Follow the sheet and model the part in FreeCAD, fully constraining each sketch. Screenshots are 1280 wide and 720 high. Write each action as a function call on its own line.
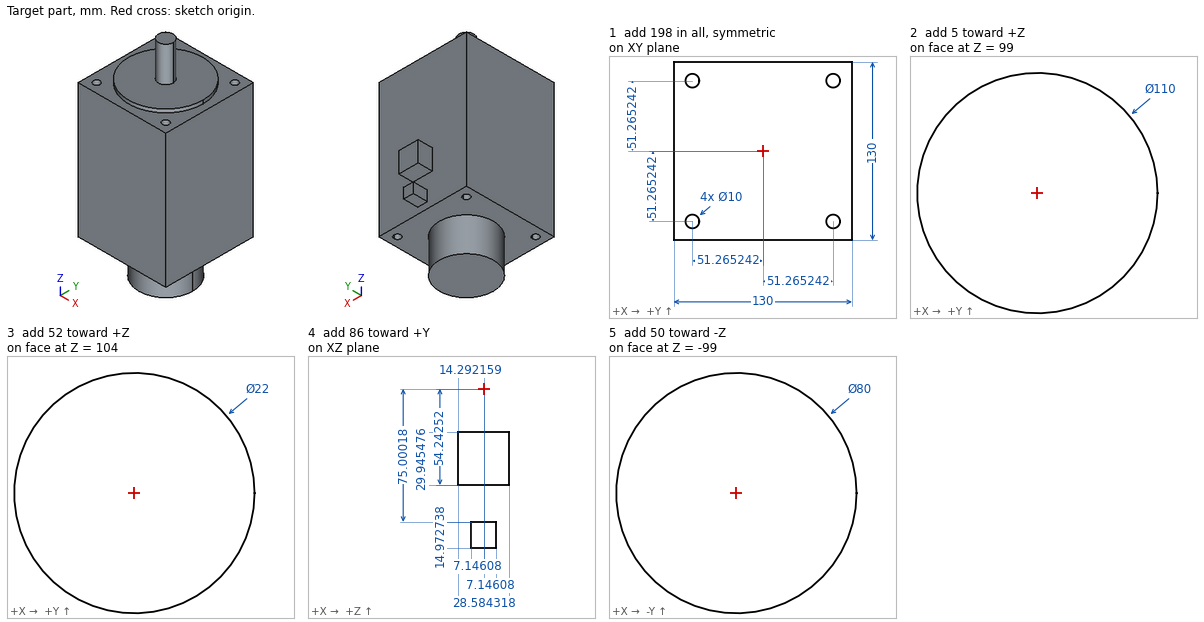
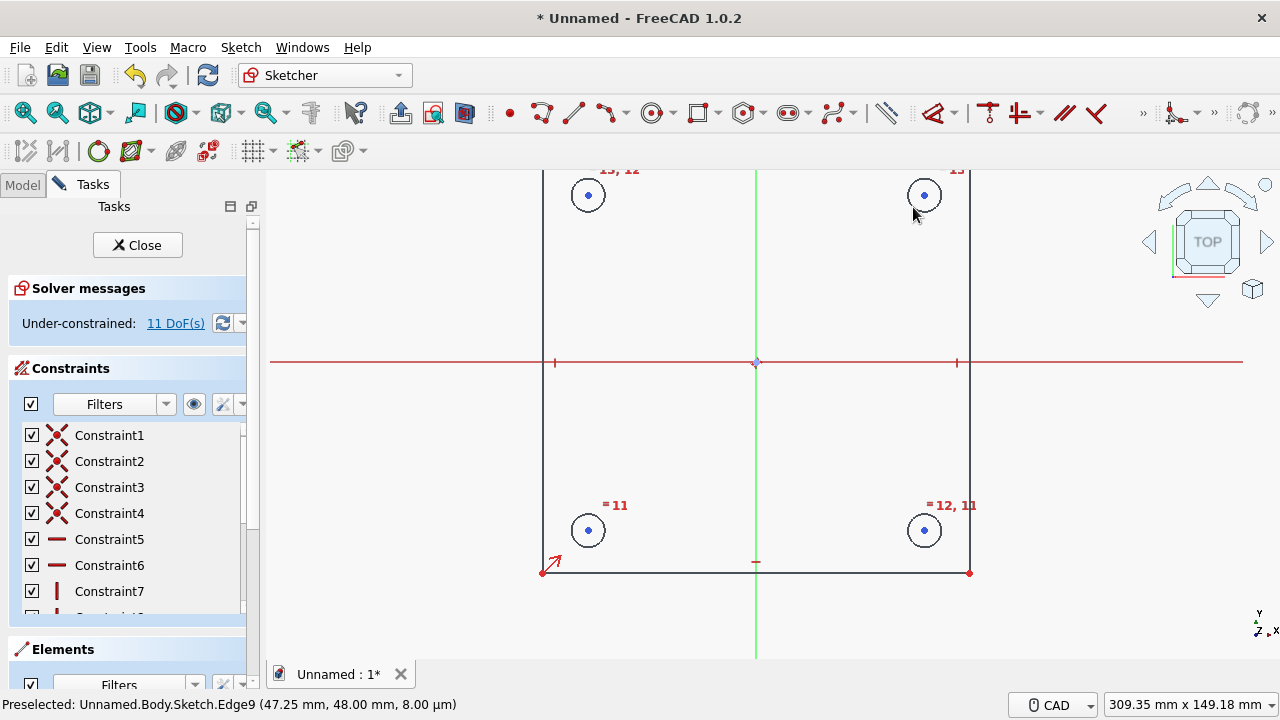
click(588, 531)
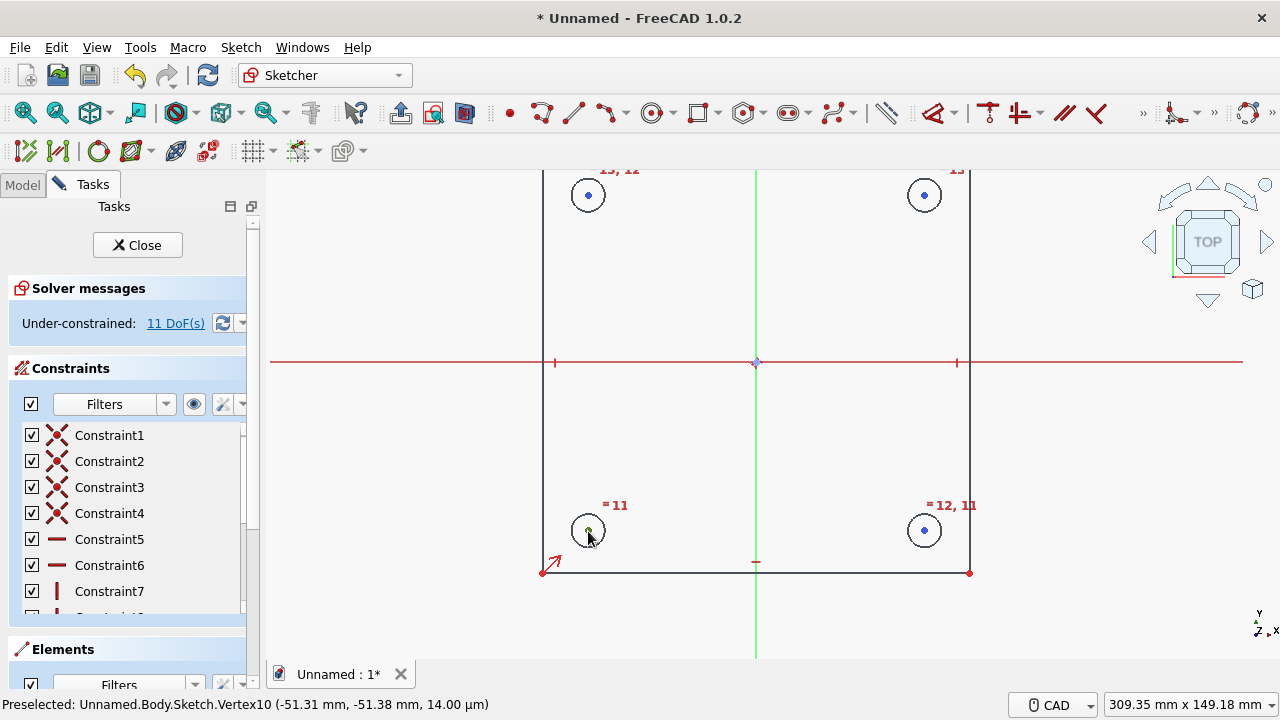
click(925, 531)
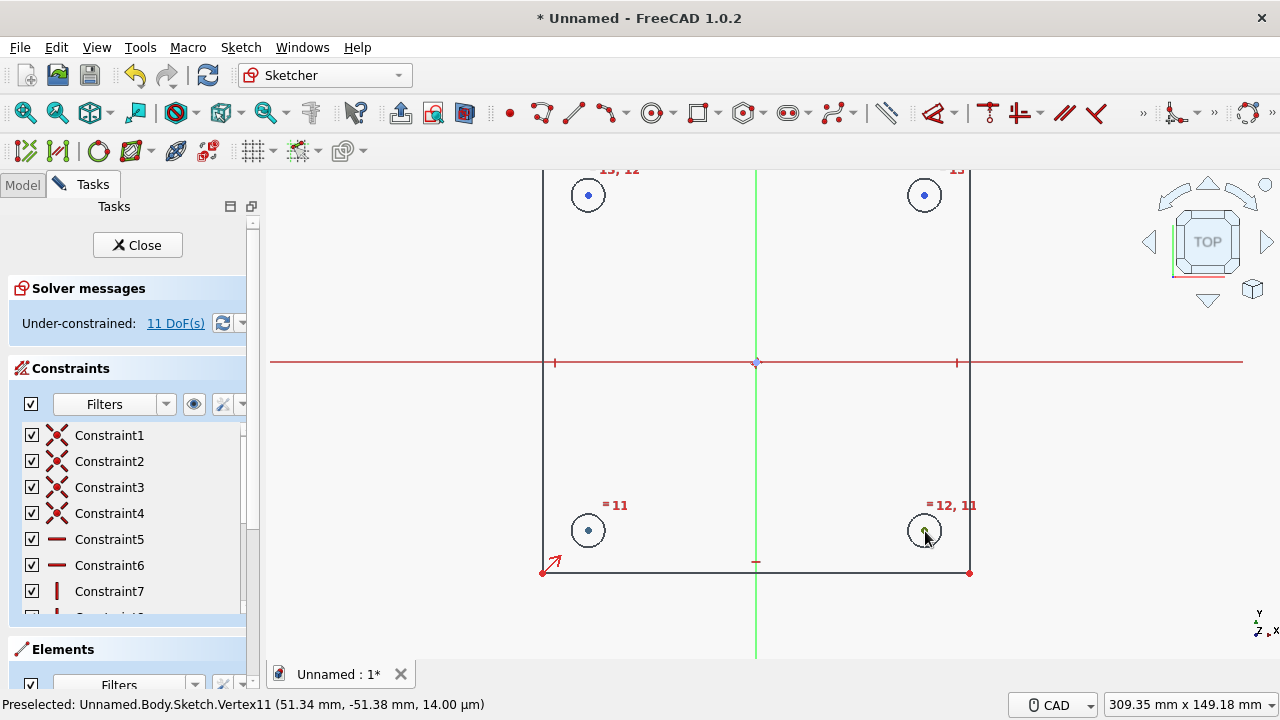
key(h)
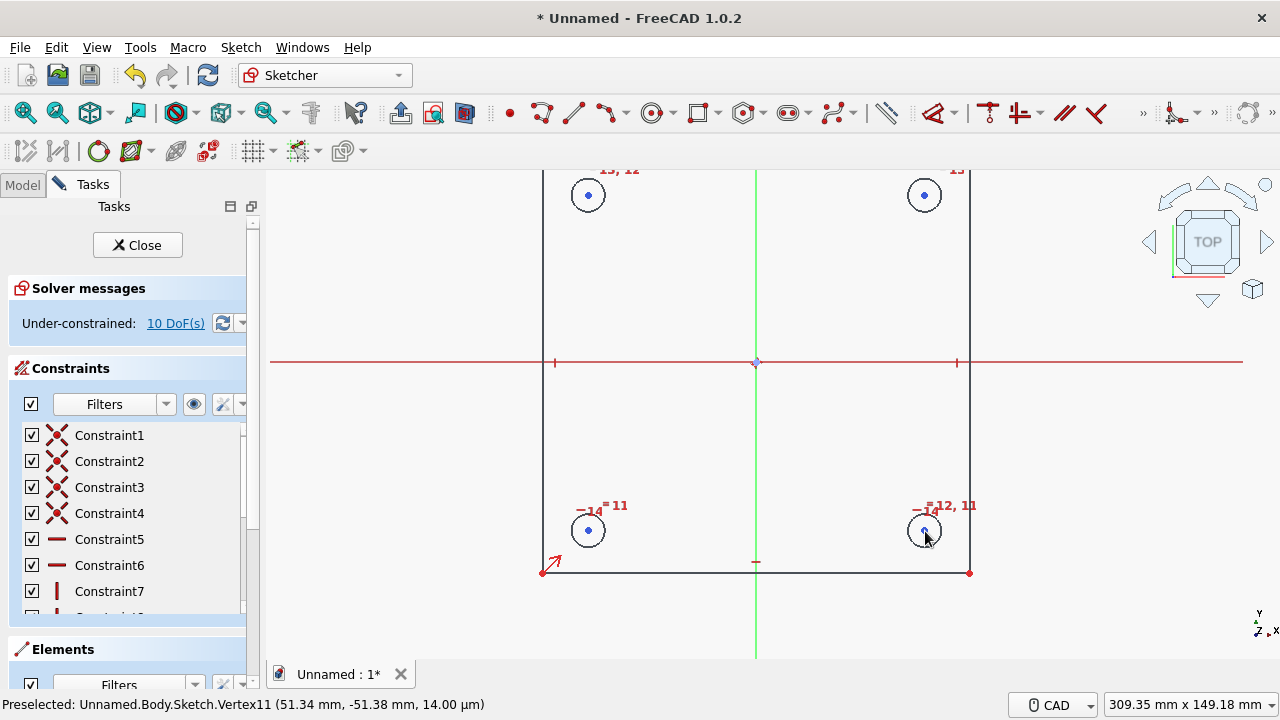
click(588, 531)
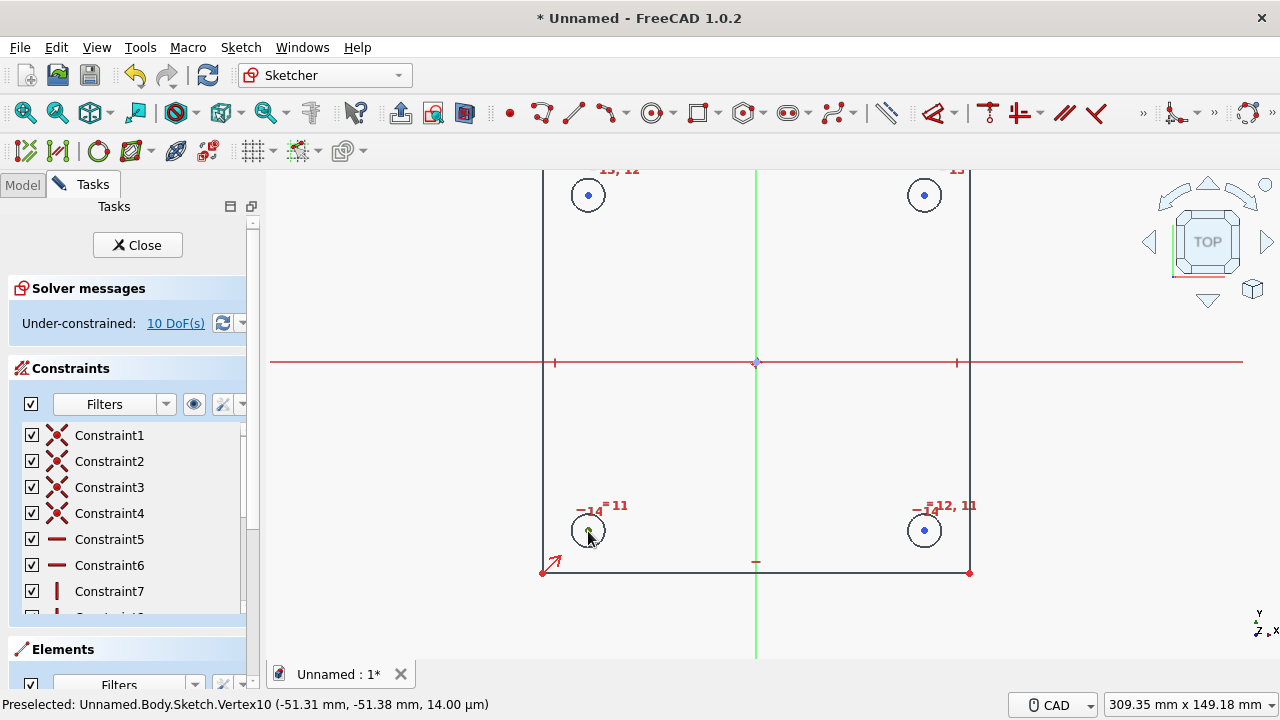
scroll(599, 521, down, 2)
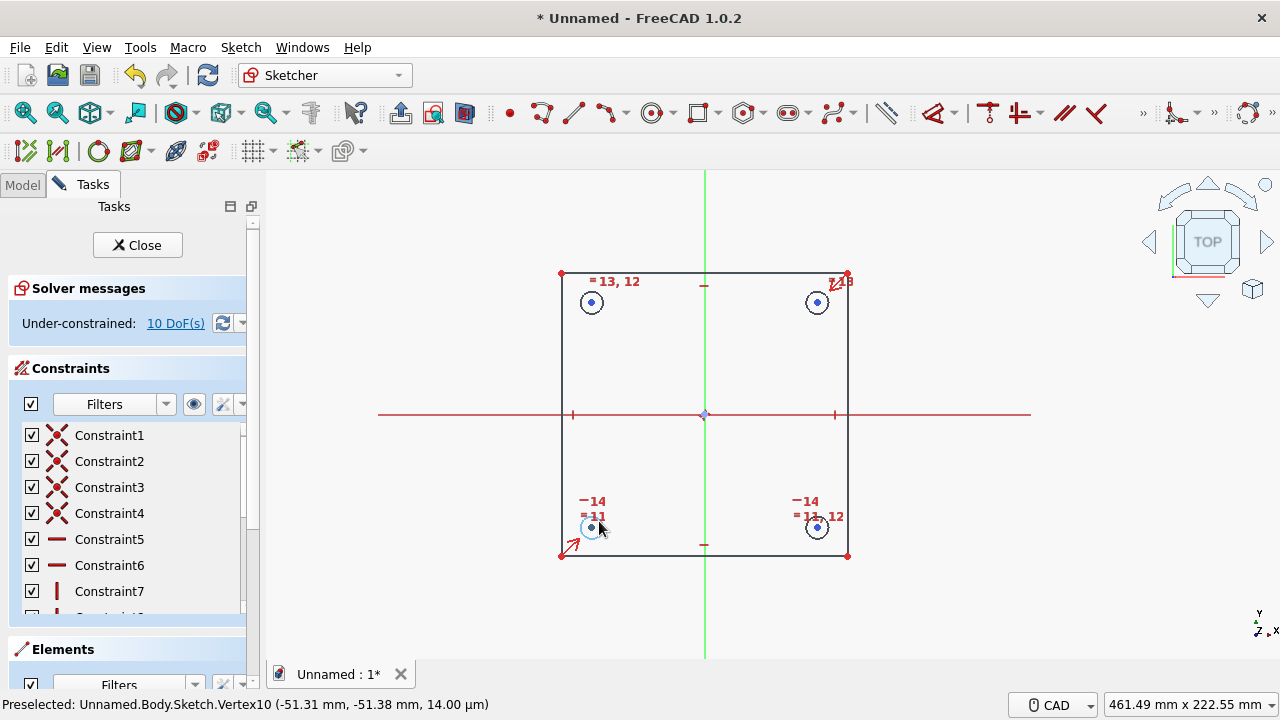
click(592, 303)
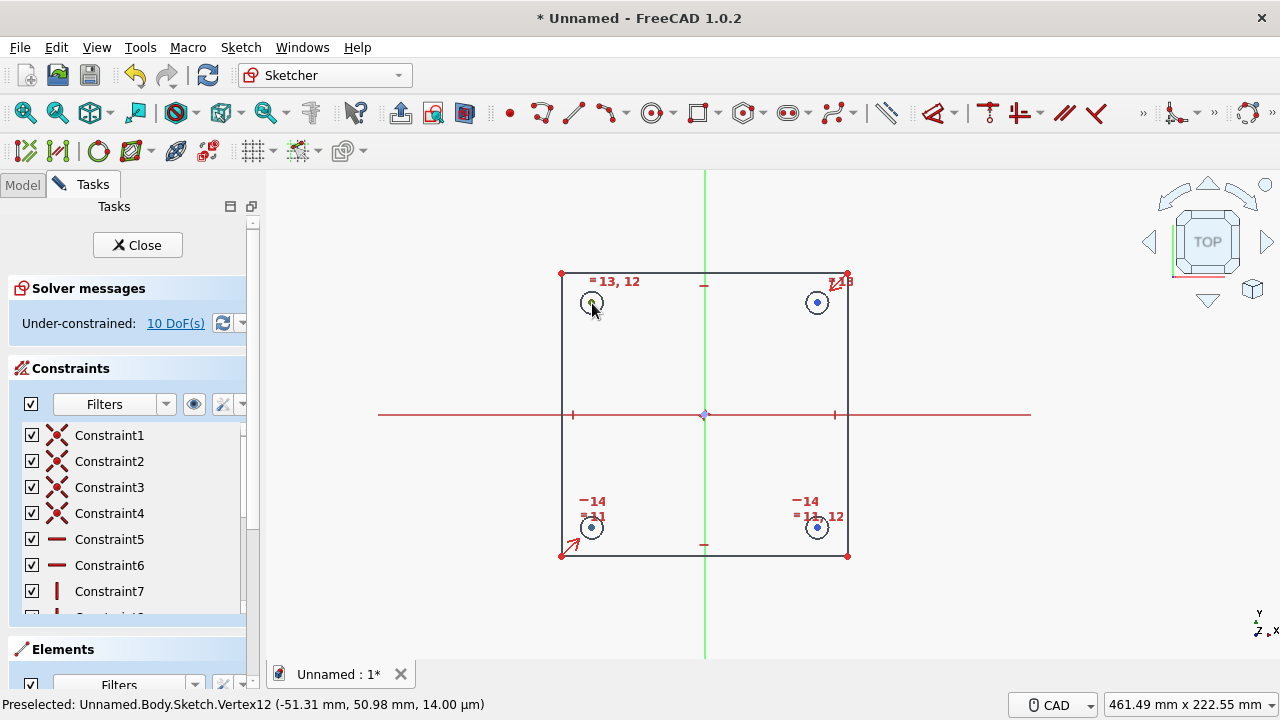
key(v)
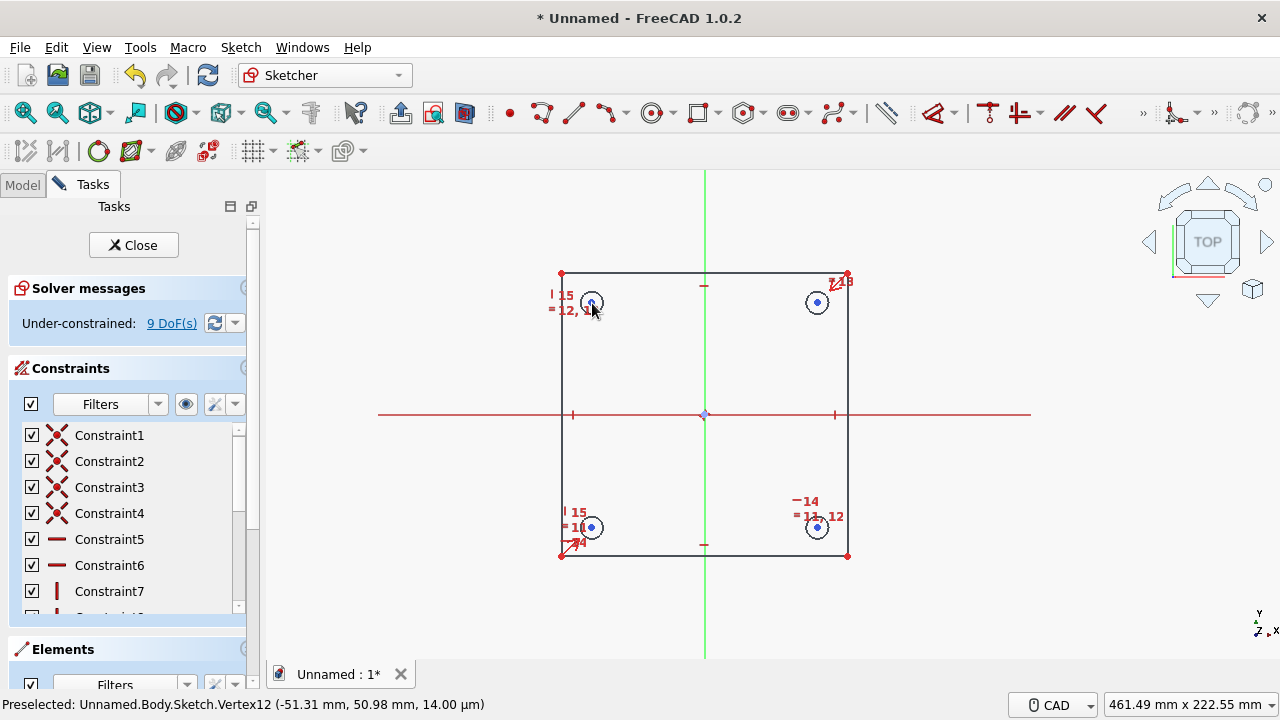
click(817, 528)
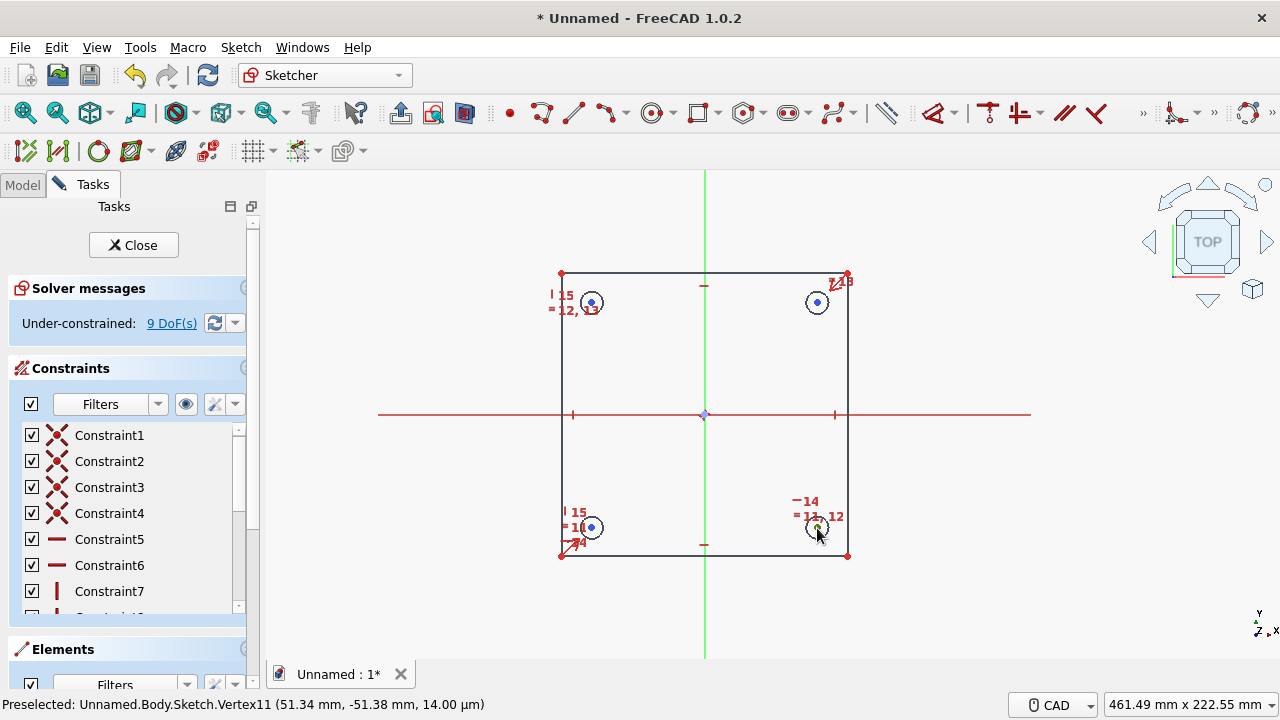
click(817, 303)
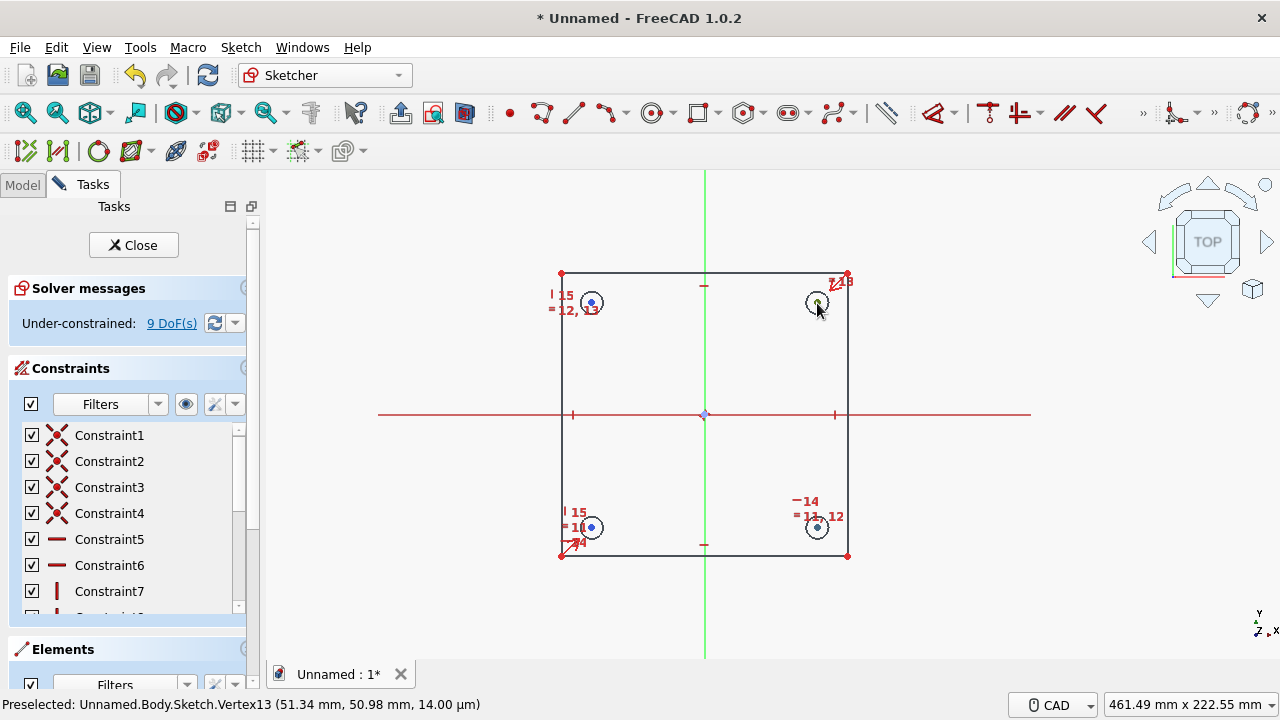
key(v)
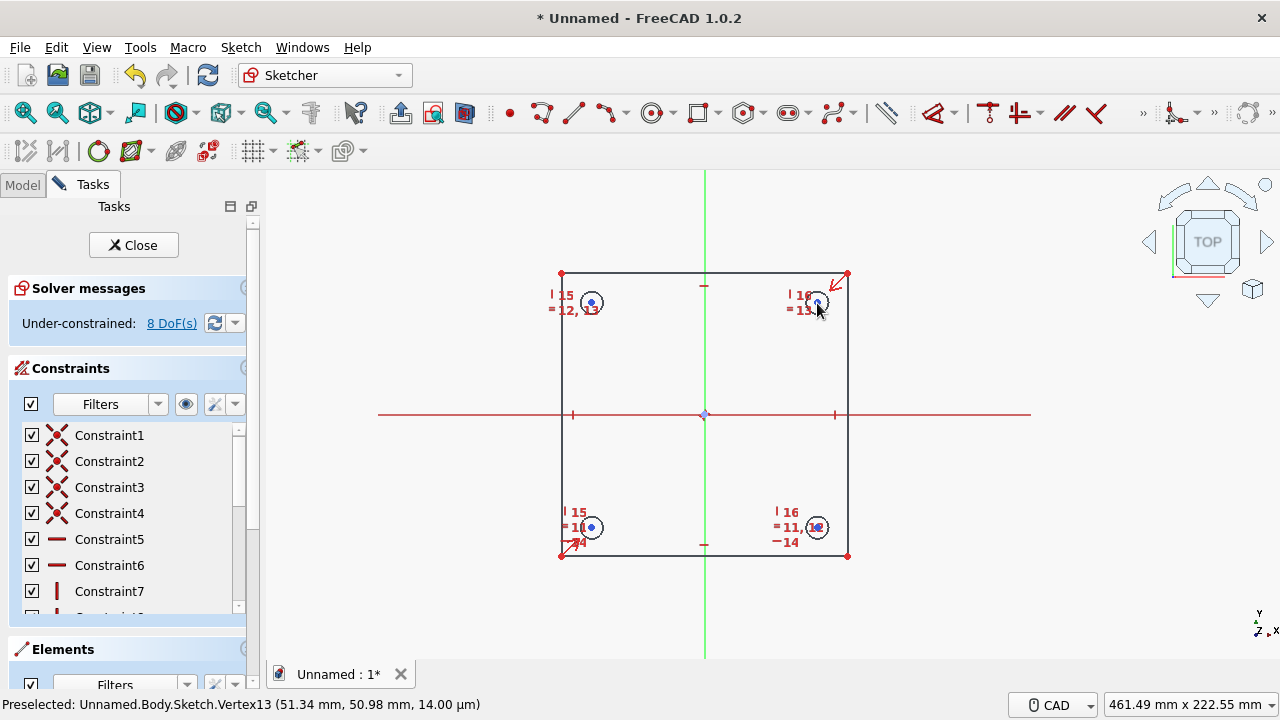
scroll(592, 303, up, 4)